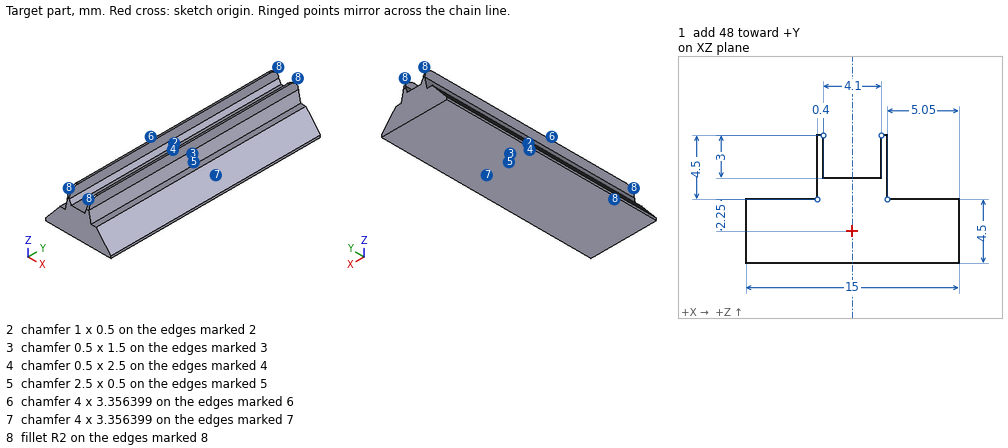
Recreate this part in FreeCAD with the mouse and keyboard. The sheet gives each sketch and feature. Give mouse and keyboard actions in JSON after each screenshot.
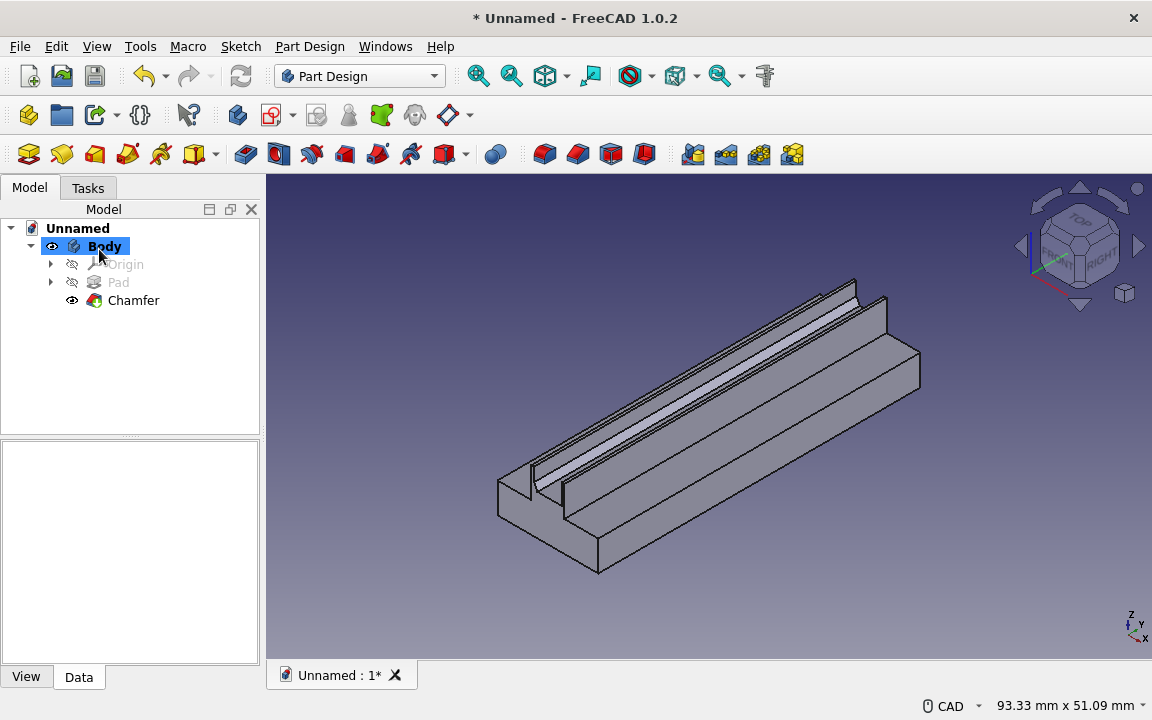
{"action": "key", "text": "1"}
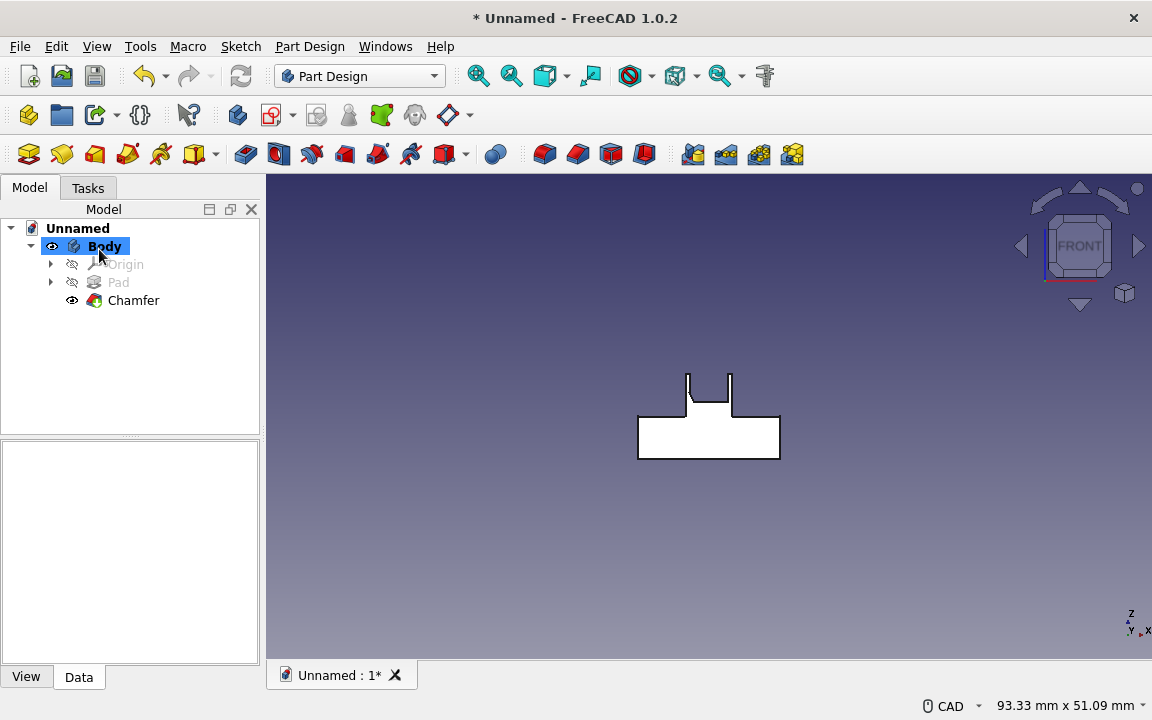
{"action": "left_click", "coordinate": [479, 76]}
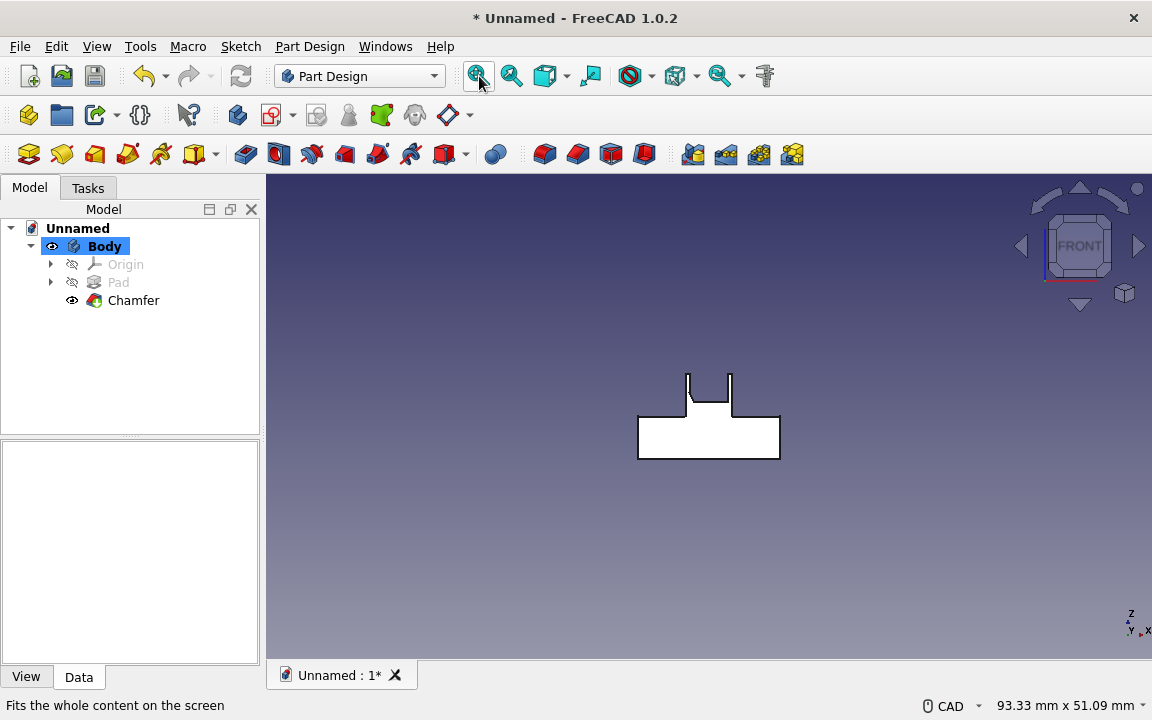
{"action": "key", "text": "3"}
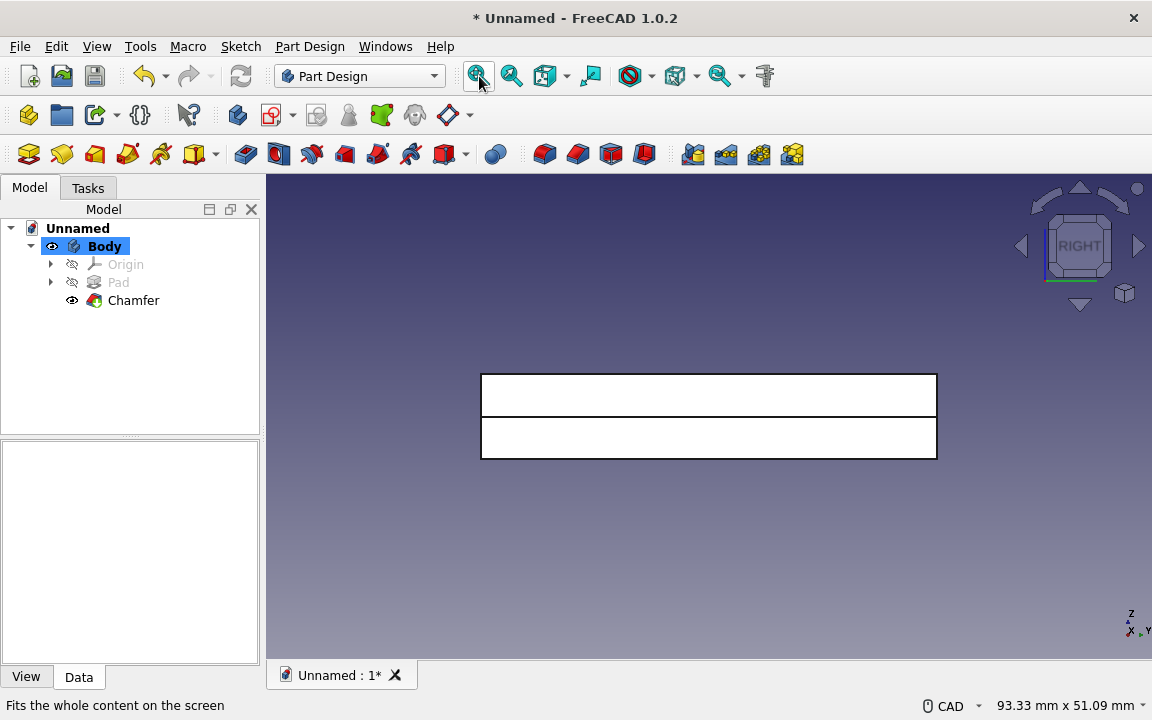
{"action": "key", "text": "5"}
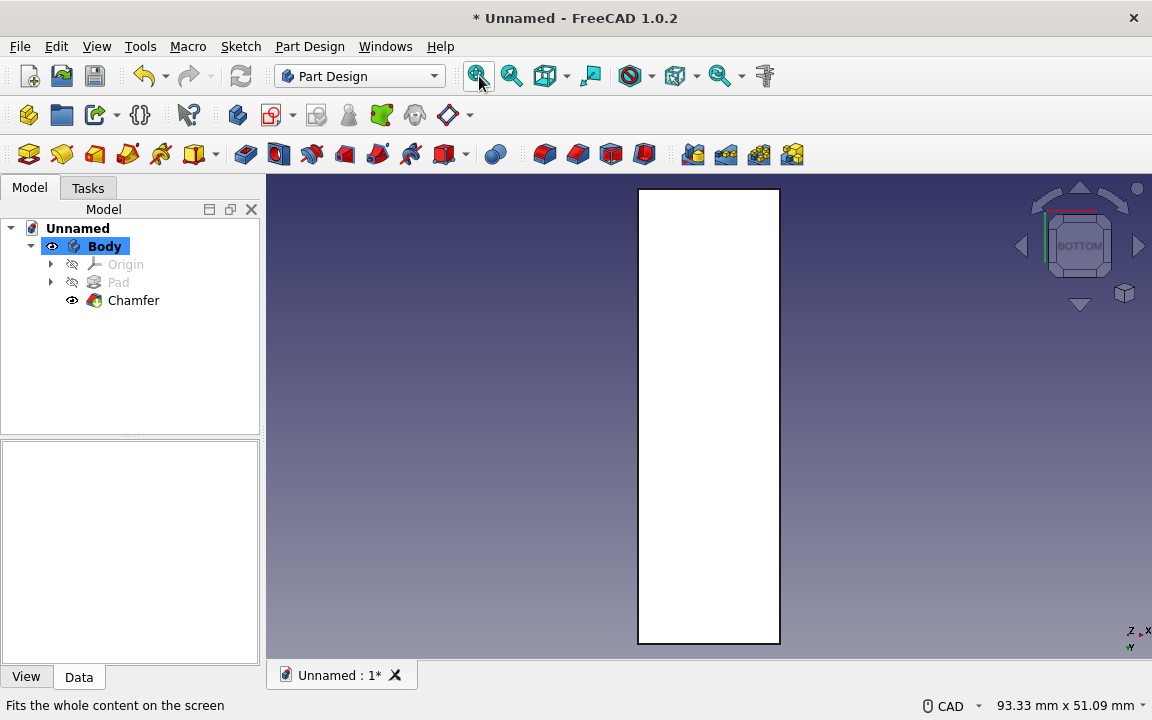
{"action": "key", "text": "4"}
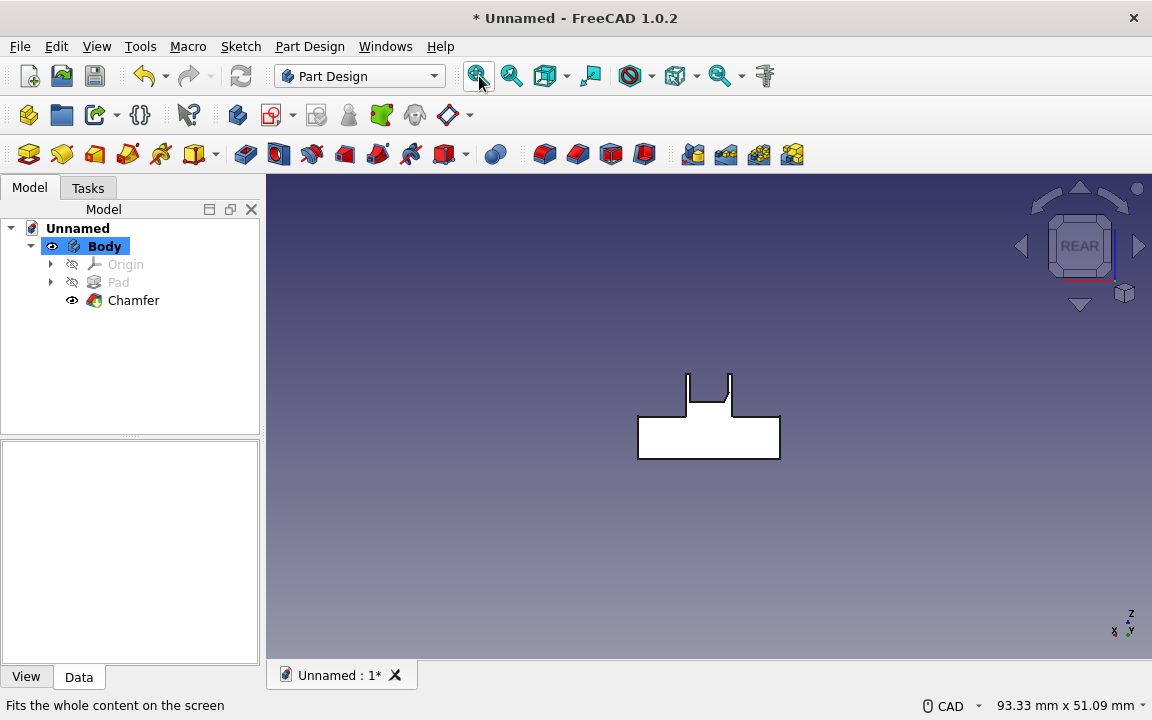
{"action": "left_click", "coordinate": [479, 76]}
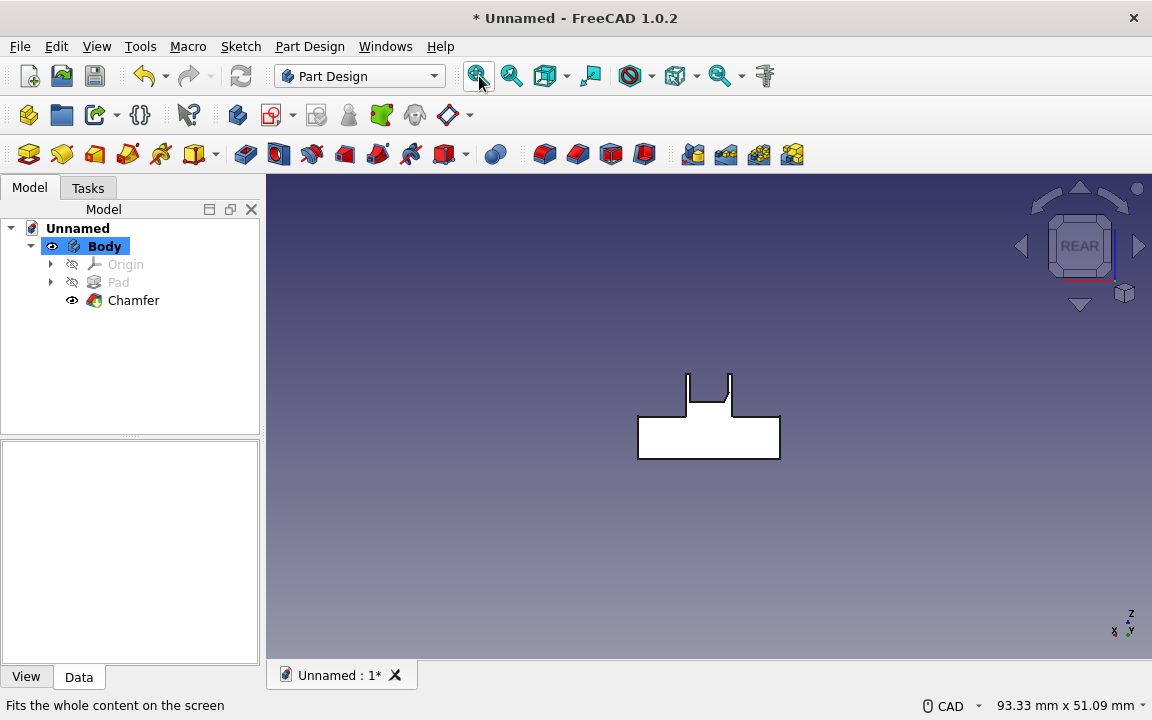
{"action": "key", "text": "6"}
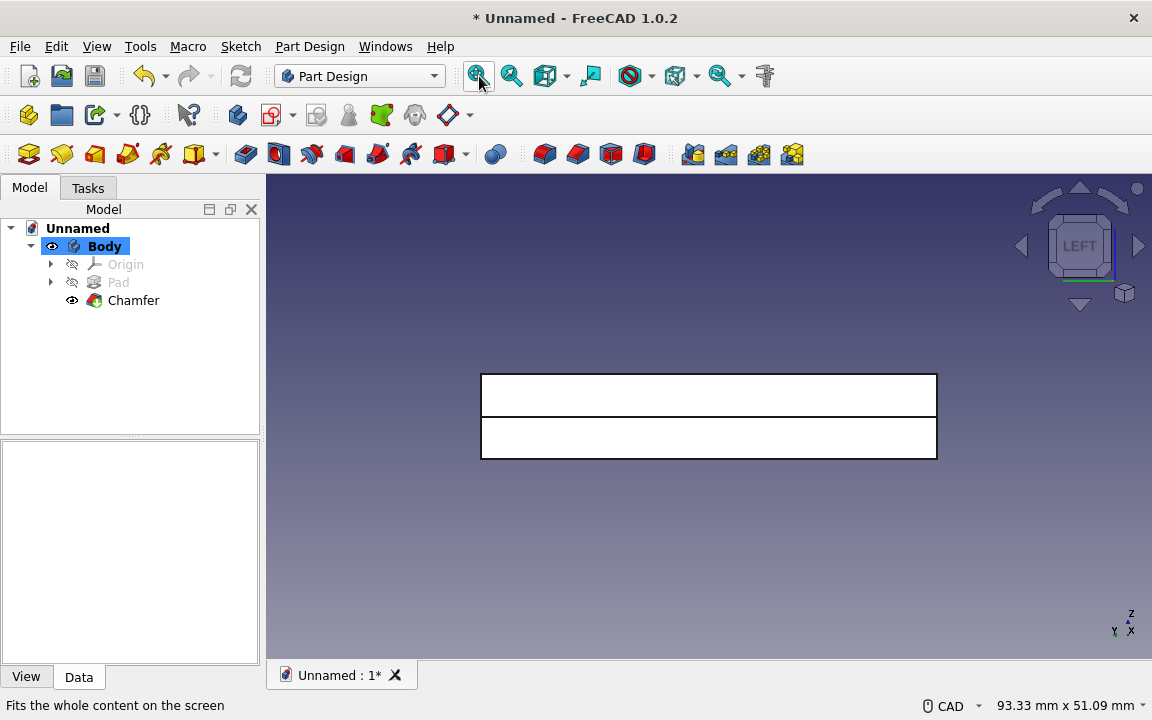
{"action": "key", "text": "v 3"}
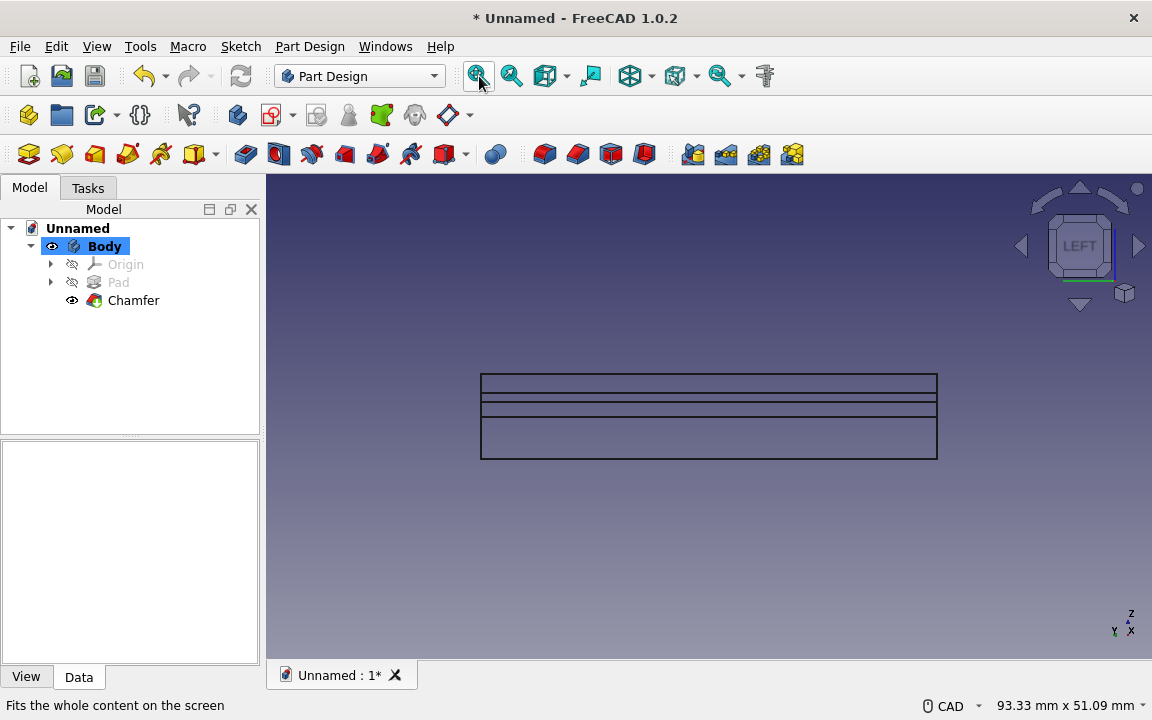
{"action": "key", "text": "0"}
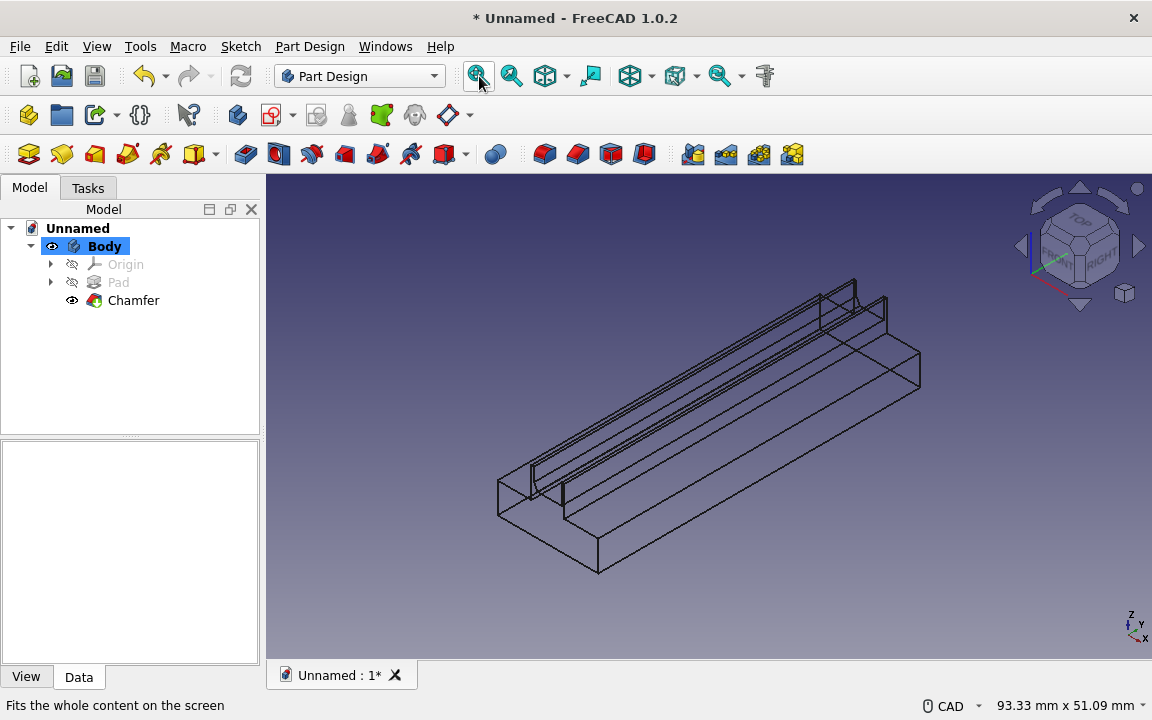
{"action": "left_click", "coordinate": [723, 412]}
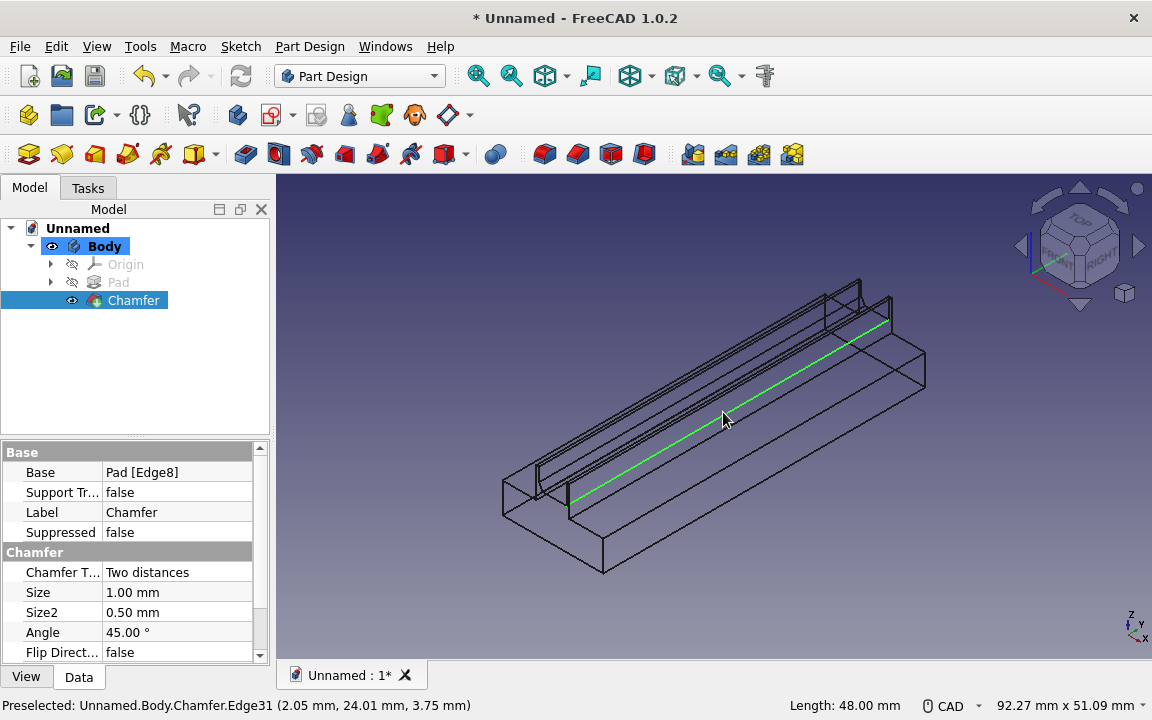
{"action": "key", "text": "v 1"}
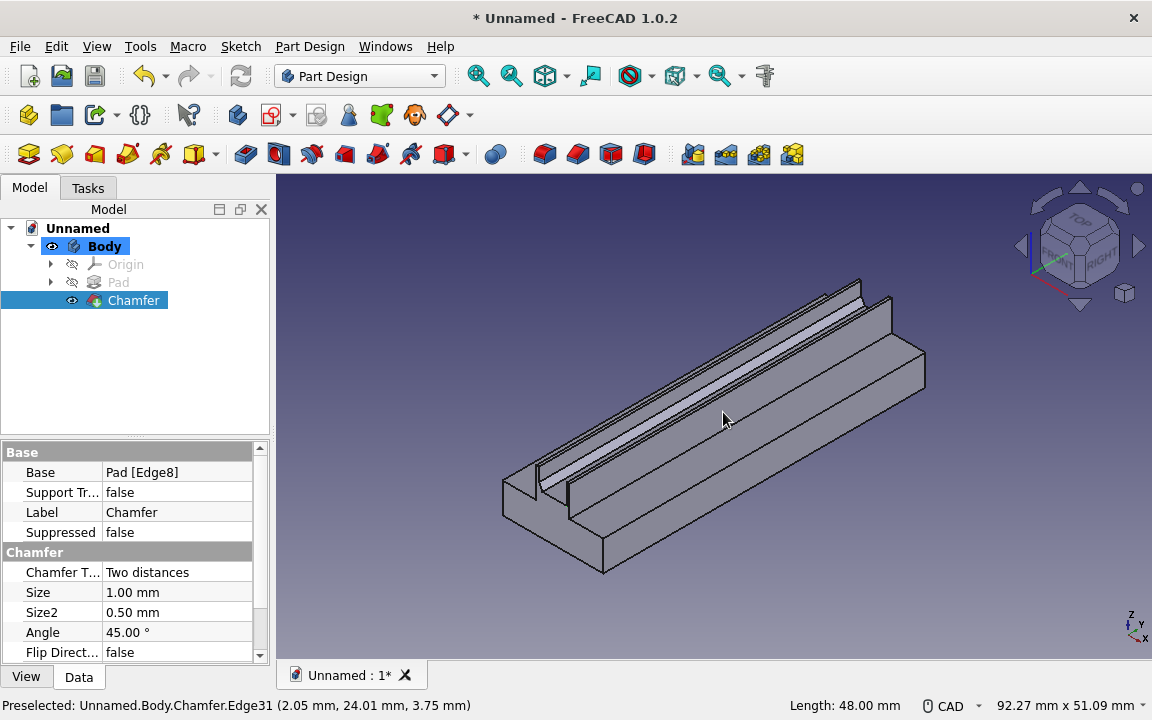
{"action": "left_click", "coordinate": [578, 154]}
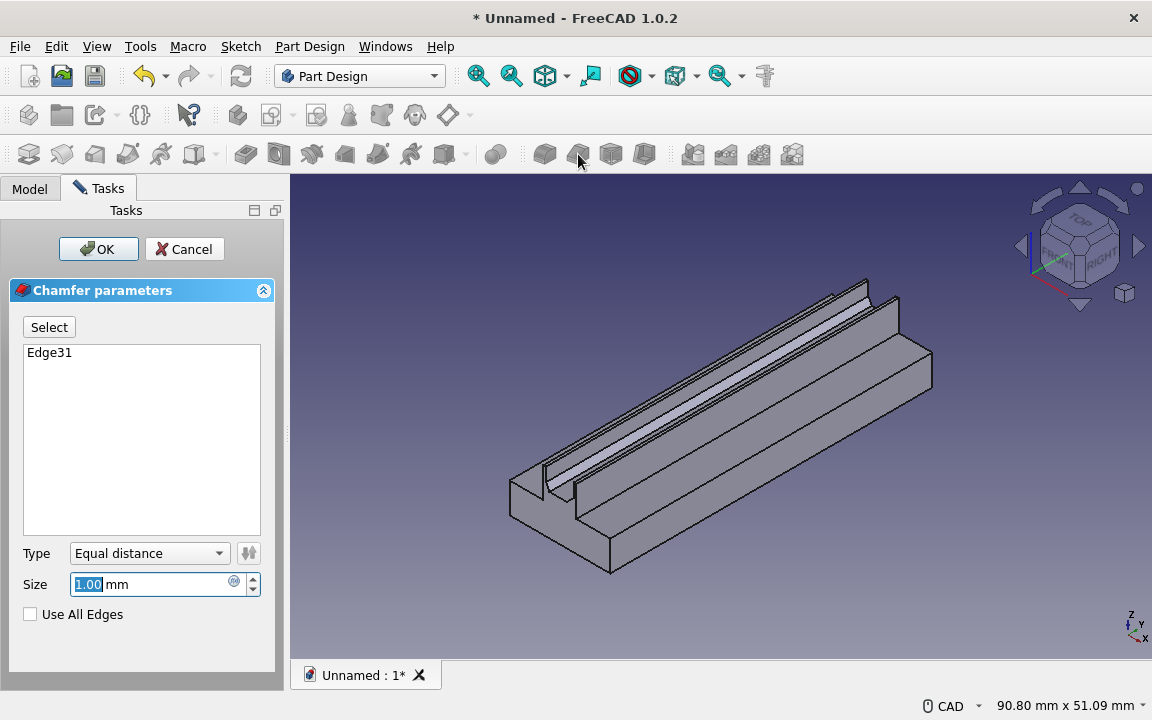
{"action": "type", "text": "0.5"}
{"action": "key", "text": "Tab"}